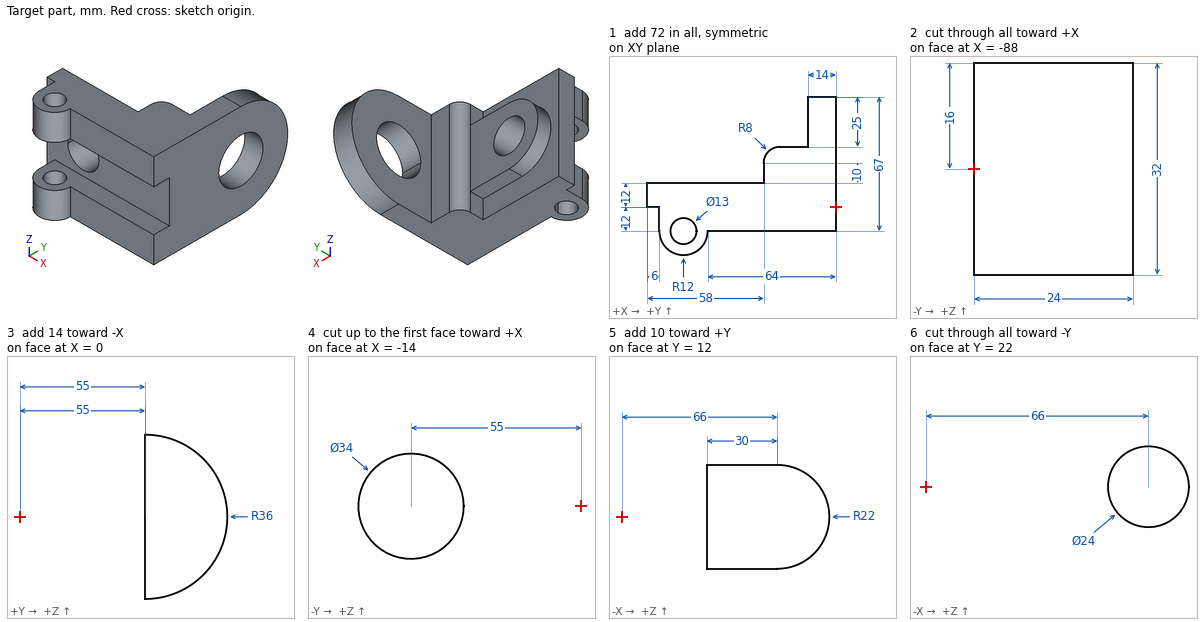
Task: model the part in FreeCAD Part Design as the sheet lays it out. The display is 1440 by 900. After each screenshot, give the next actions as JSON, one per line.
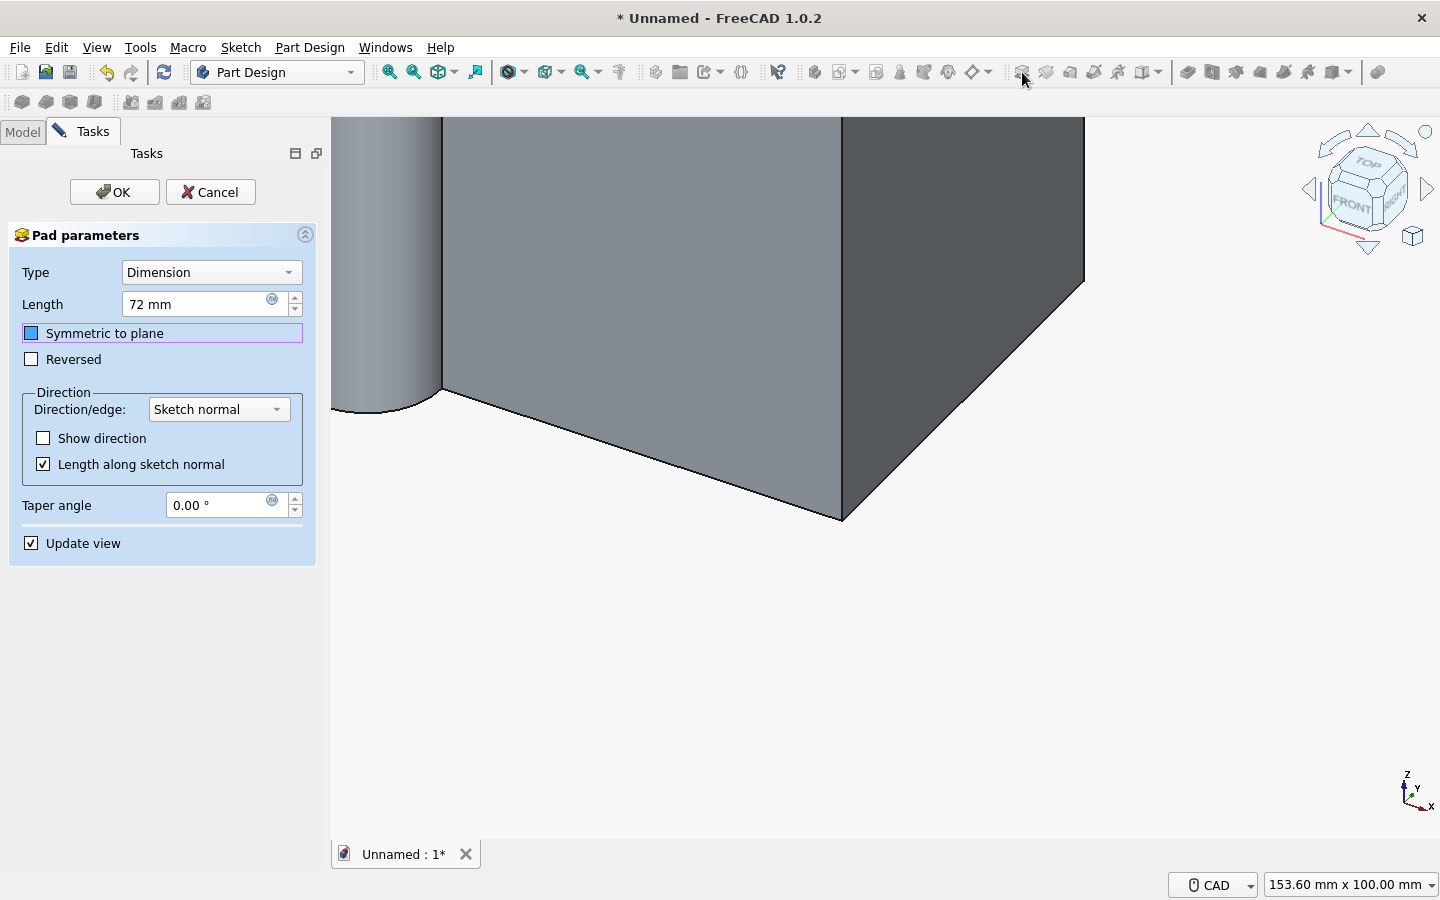
{"action": "left_click", "coordinate": [30, 333]}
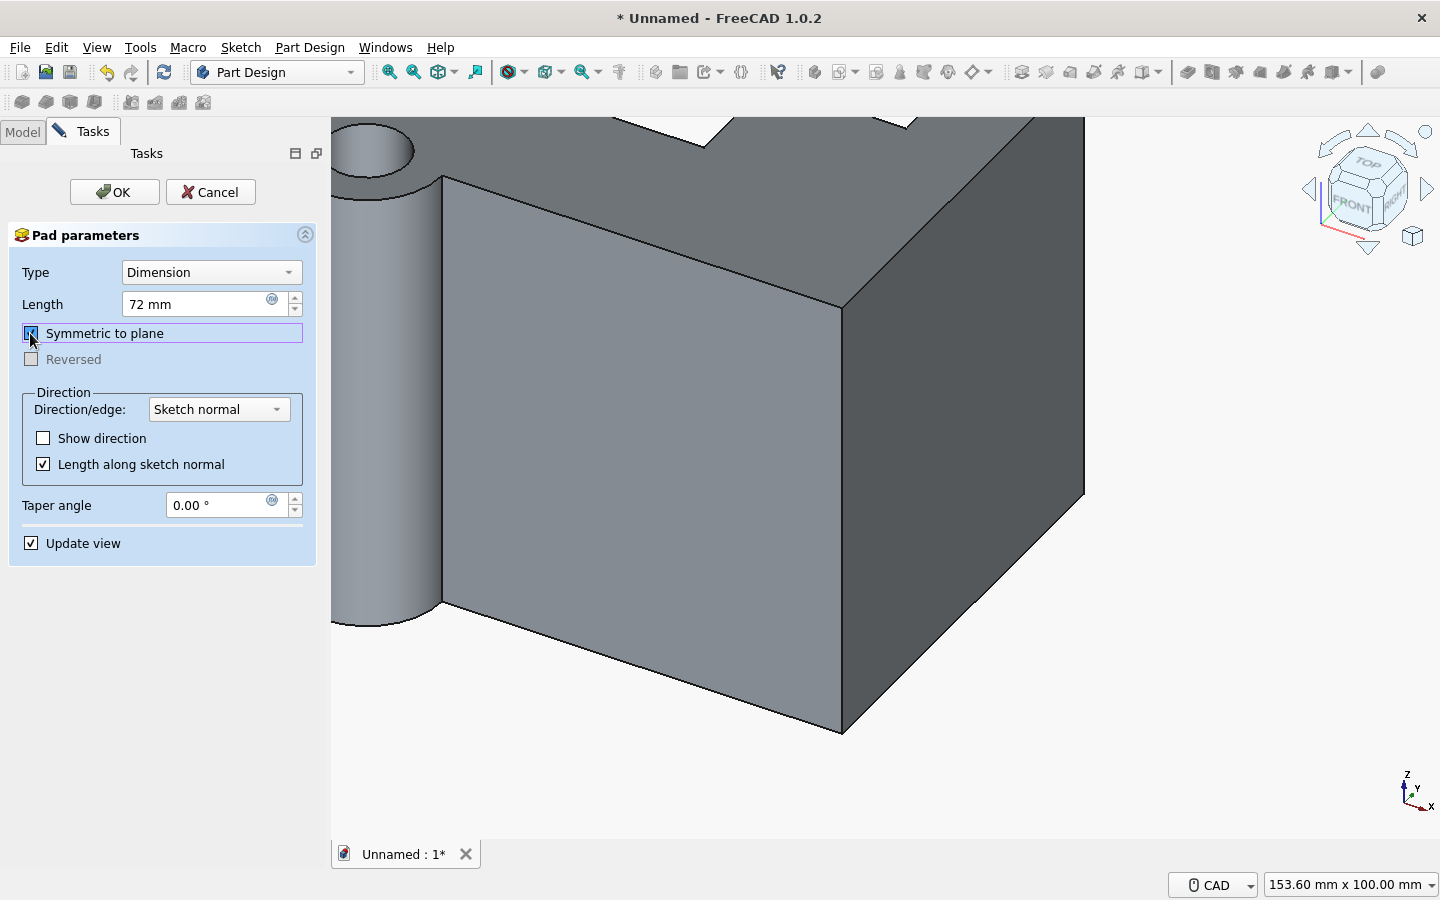
{"action": "left_click", "coordinate": [115, 192]}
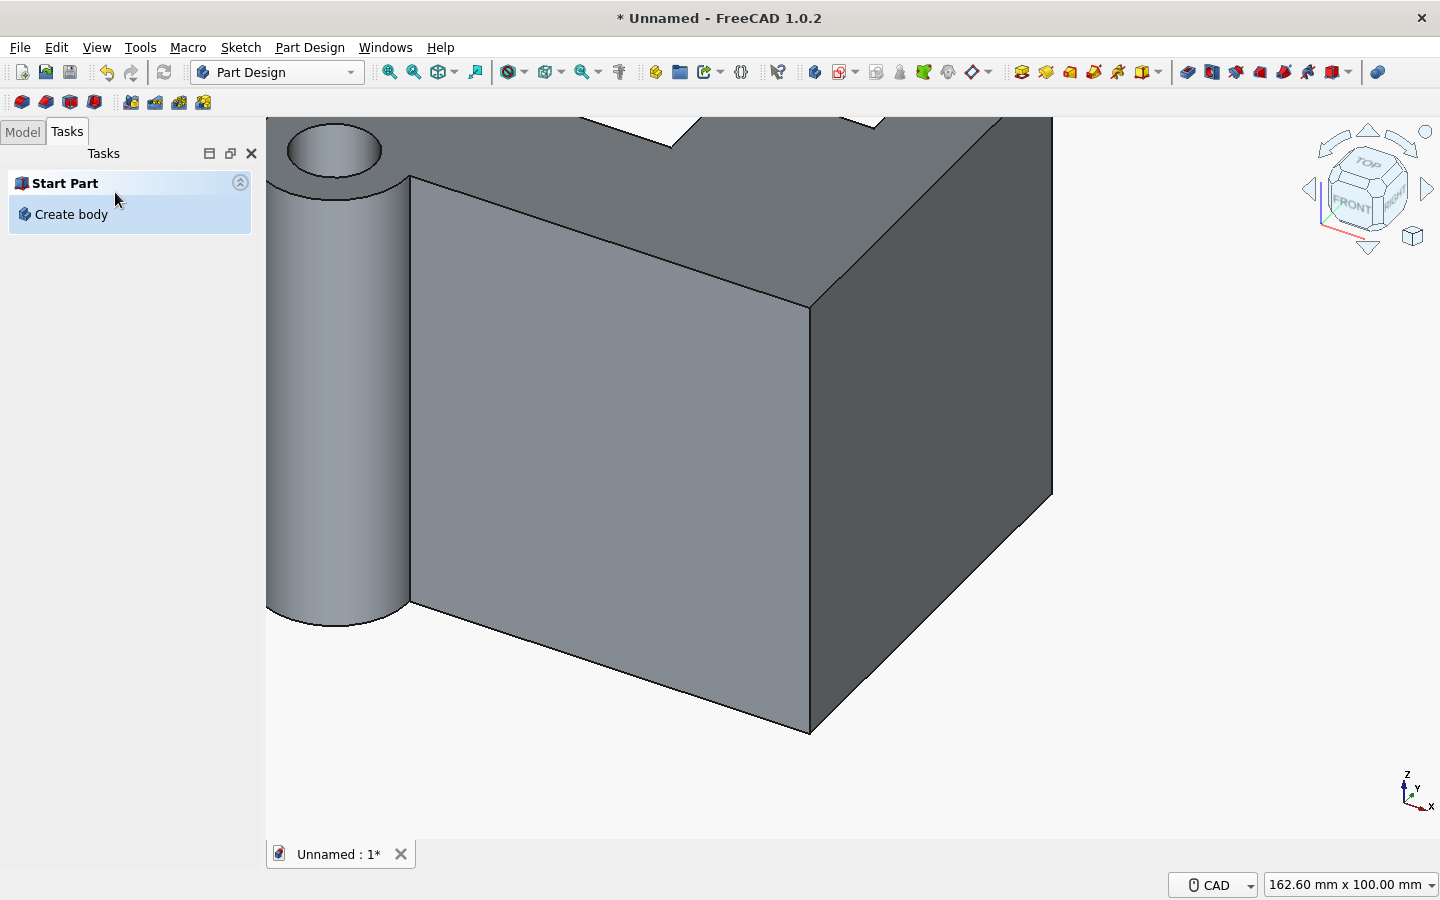
{"action": "left_click", "coordinate": [390, 72]}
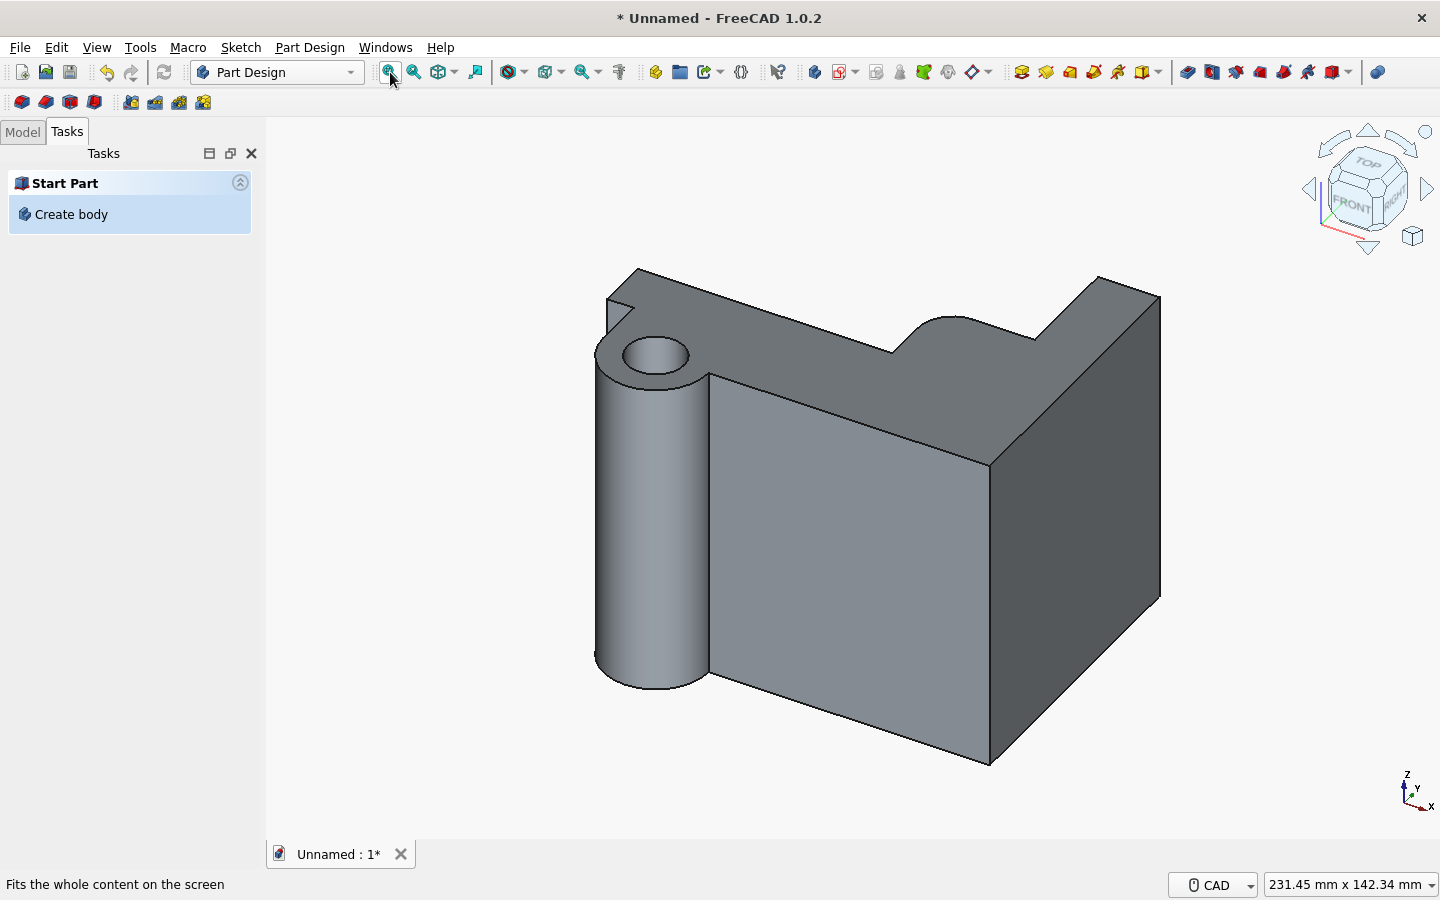
{"action": "key", "text": "6"}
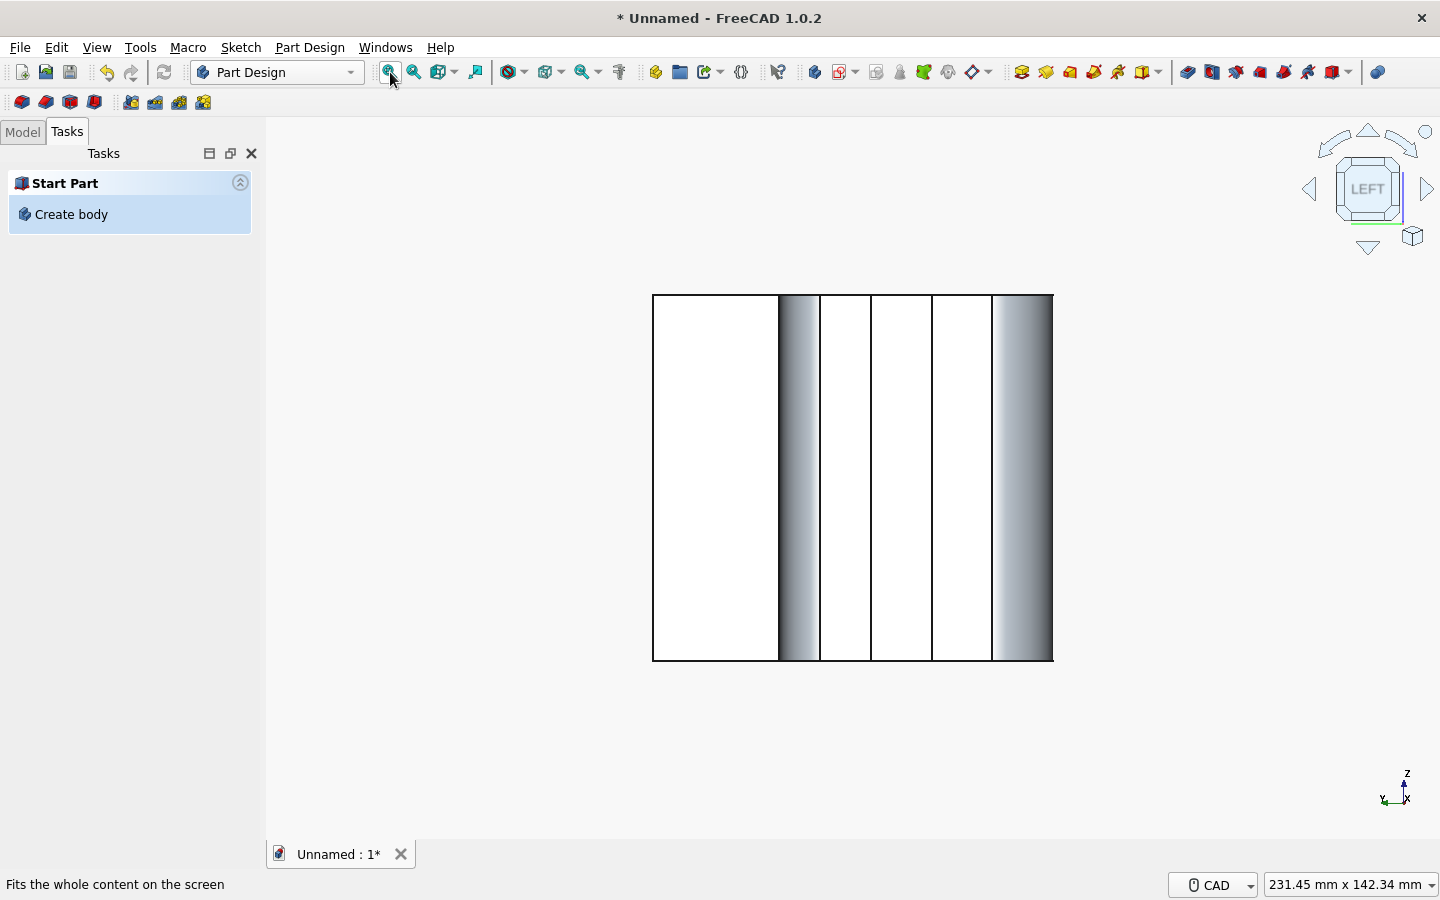
{"action": "left_click", "coordinate": [962, 373]}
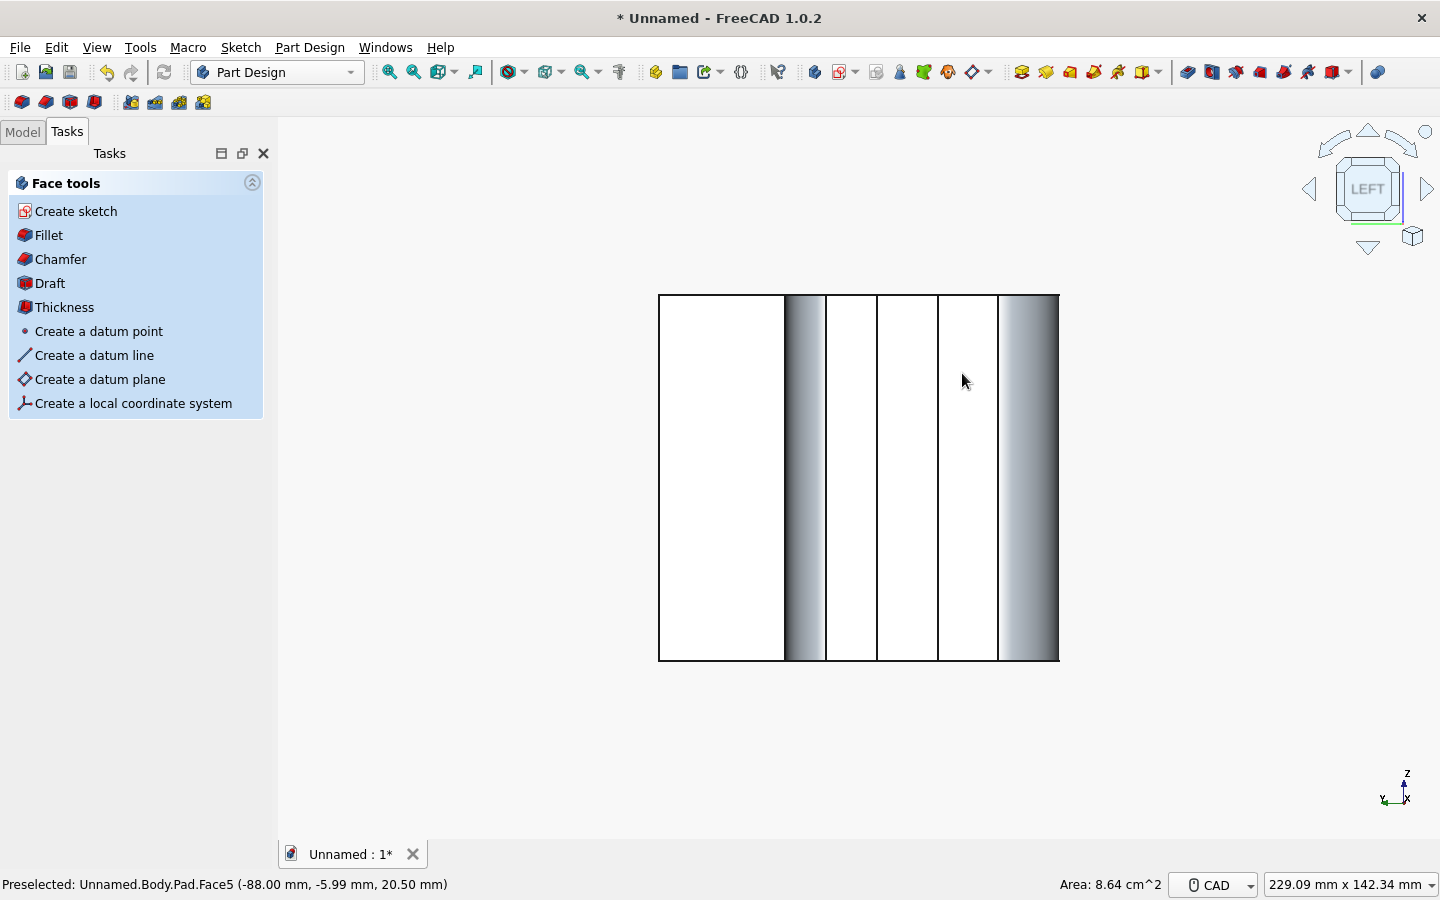
{"action": "left_click", "coordinate": [840, 72]}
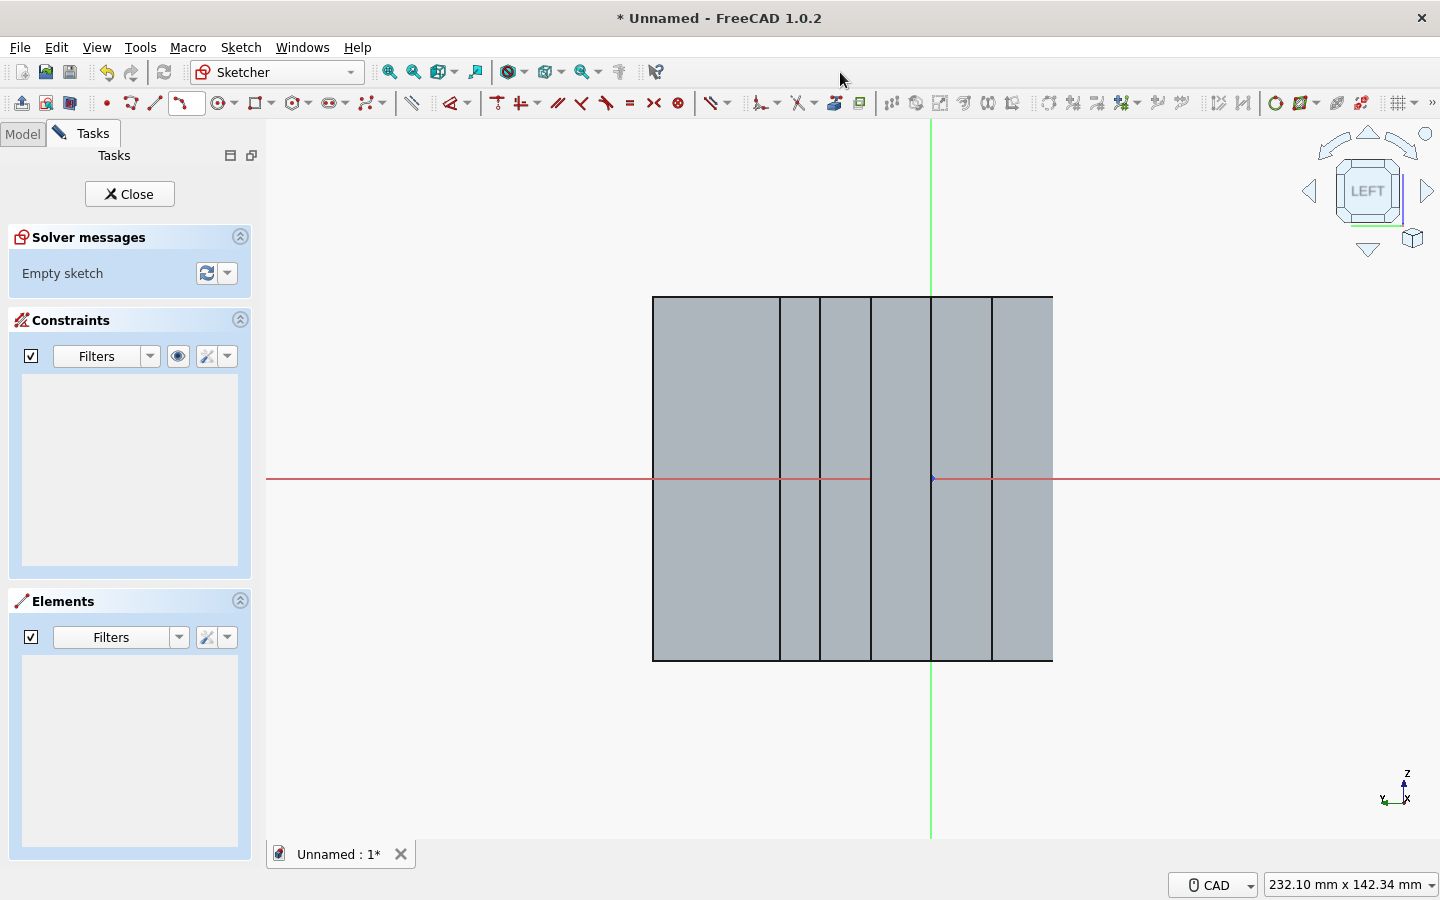
{"action": "left_click", "coordinate": [70, 104]}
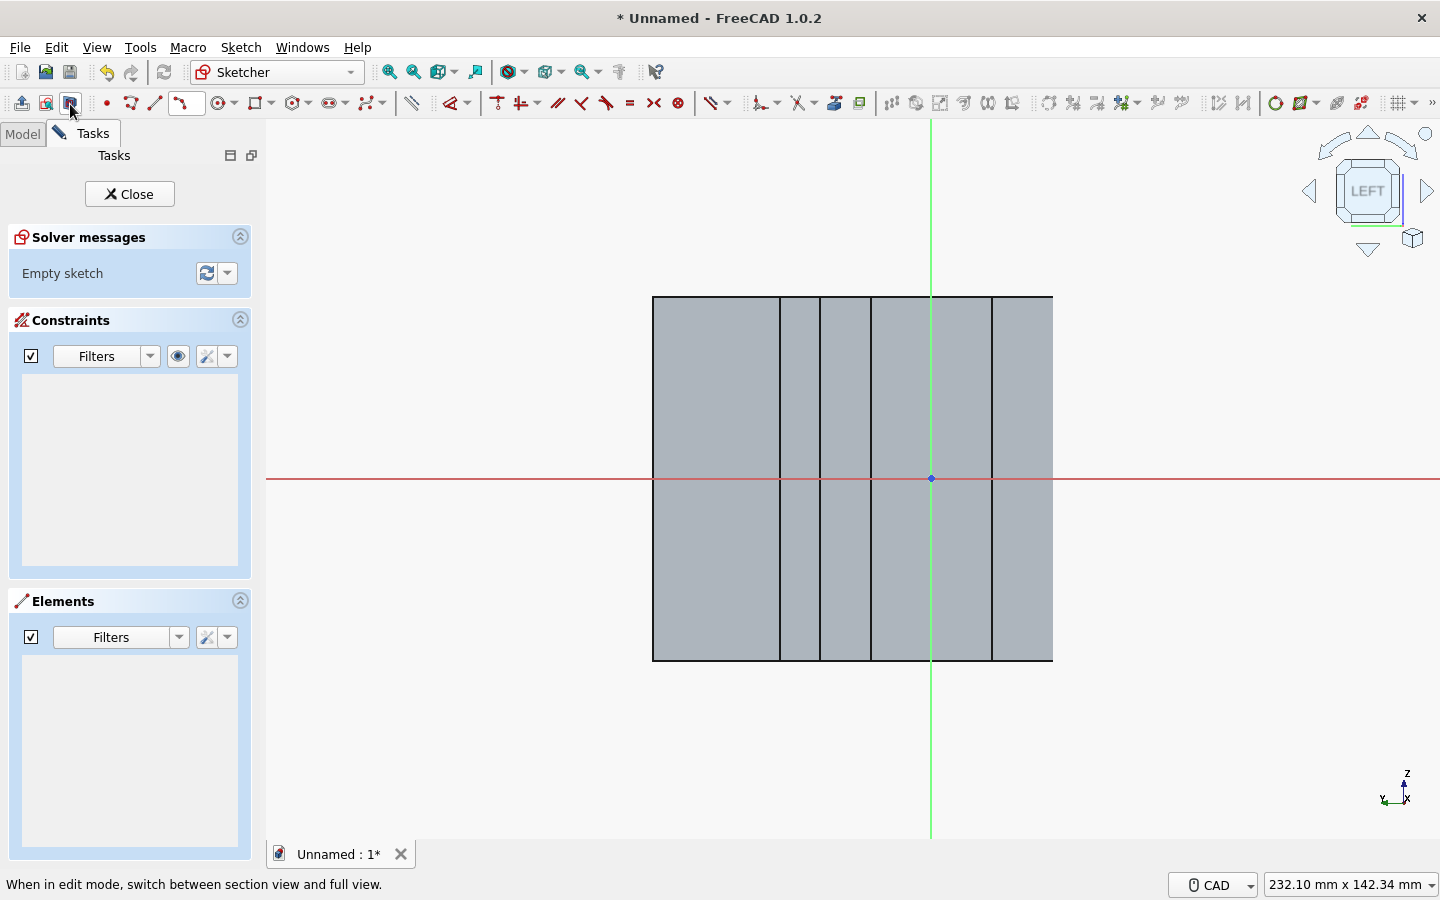
{"action": "scroll", "coordinate": [1113, 479], "scroll_direction": "up", "scroll_amount": 5}